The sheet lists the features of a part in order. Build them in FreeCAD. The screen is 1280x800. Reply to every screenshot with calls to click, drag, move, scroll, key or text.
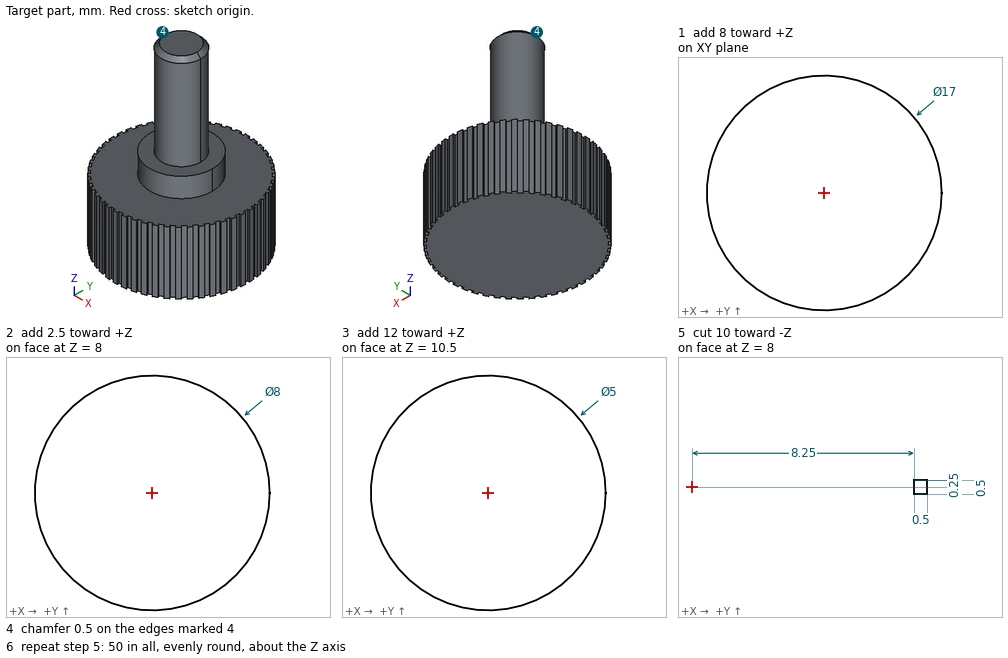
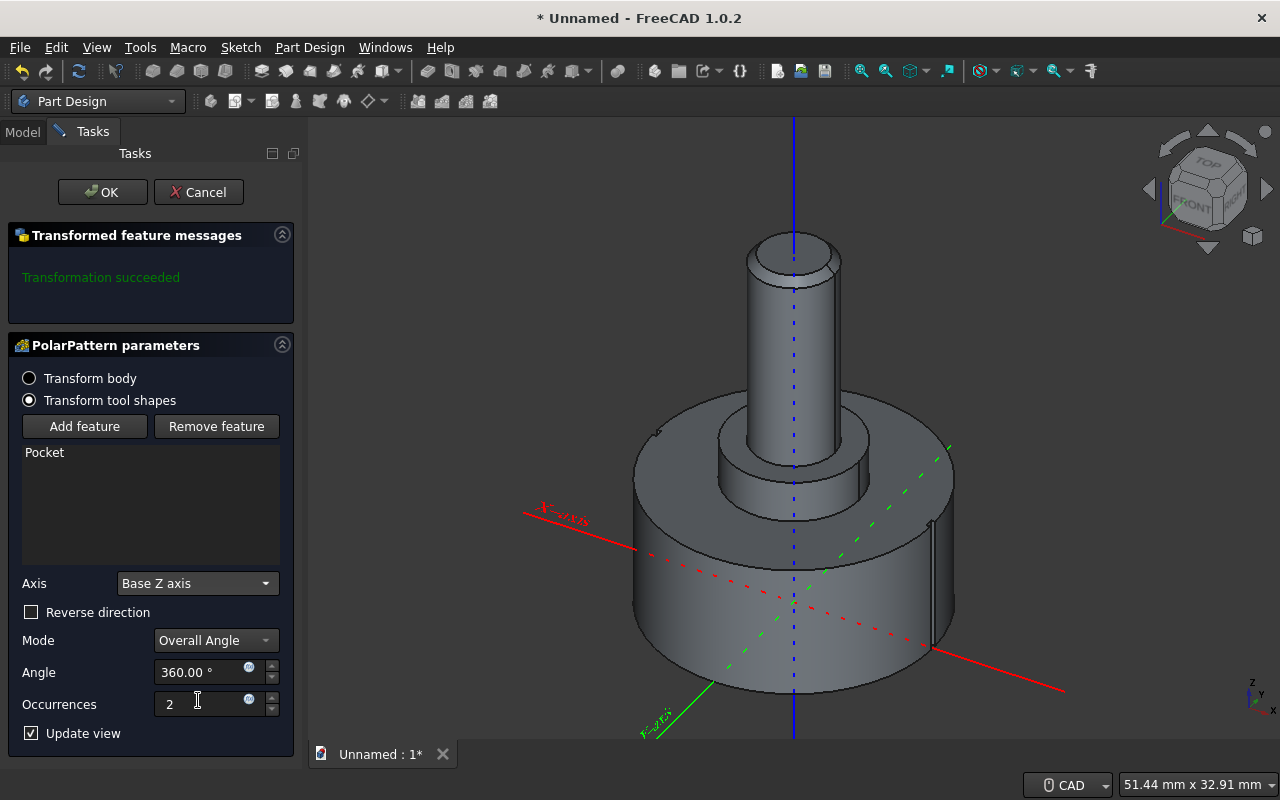
triple_click(209, 704)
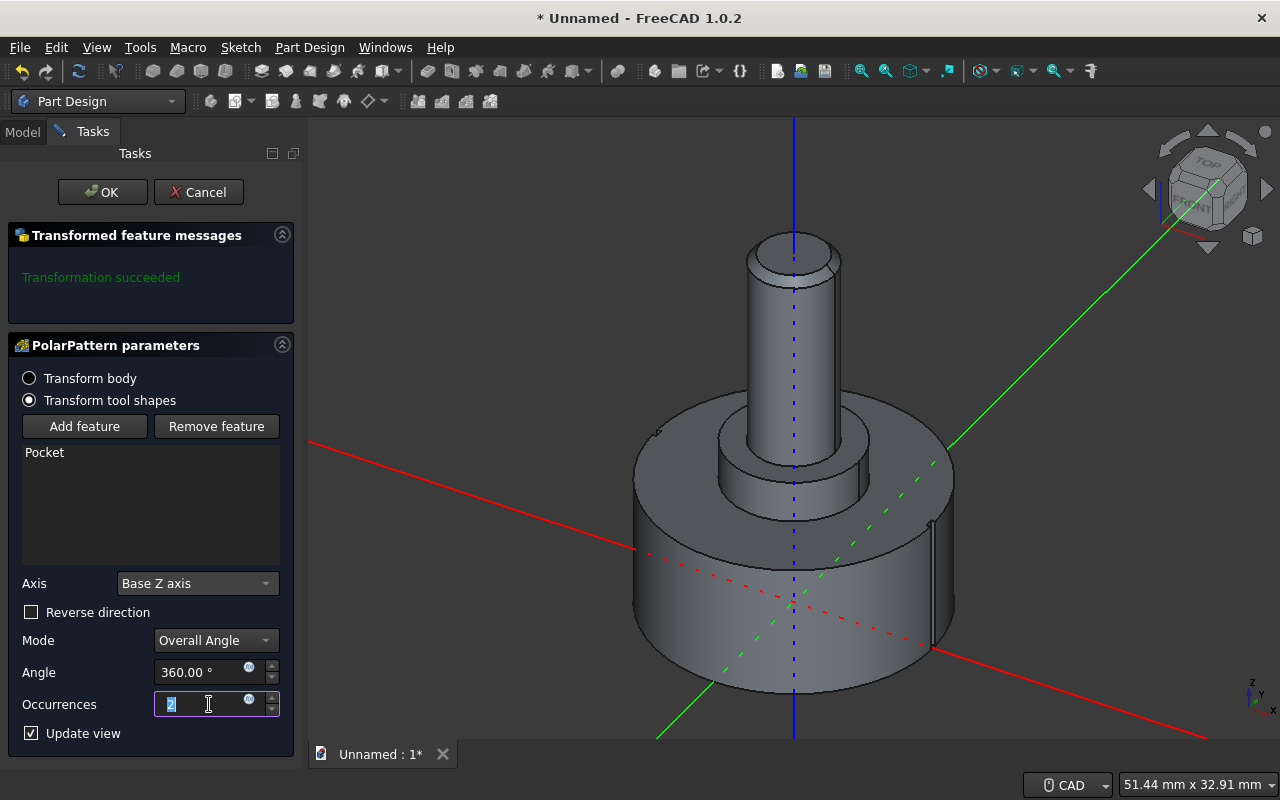
text(50)
key(Tab)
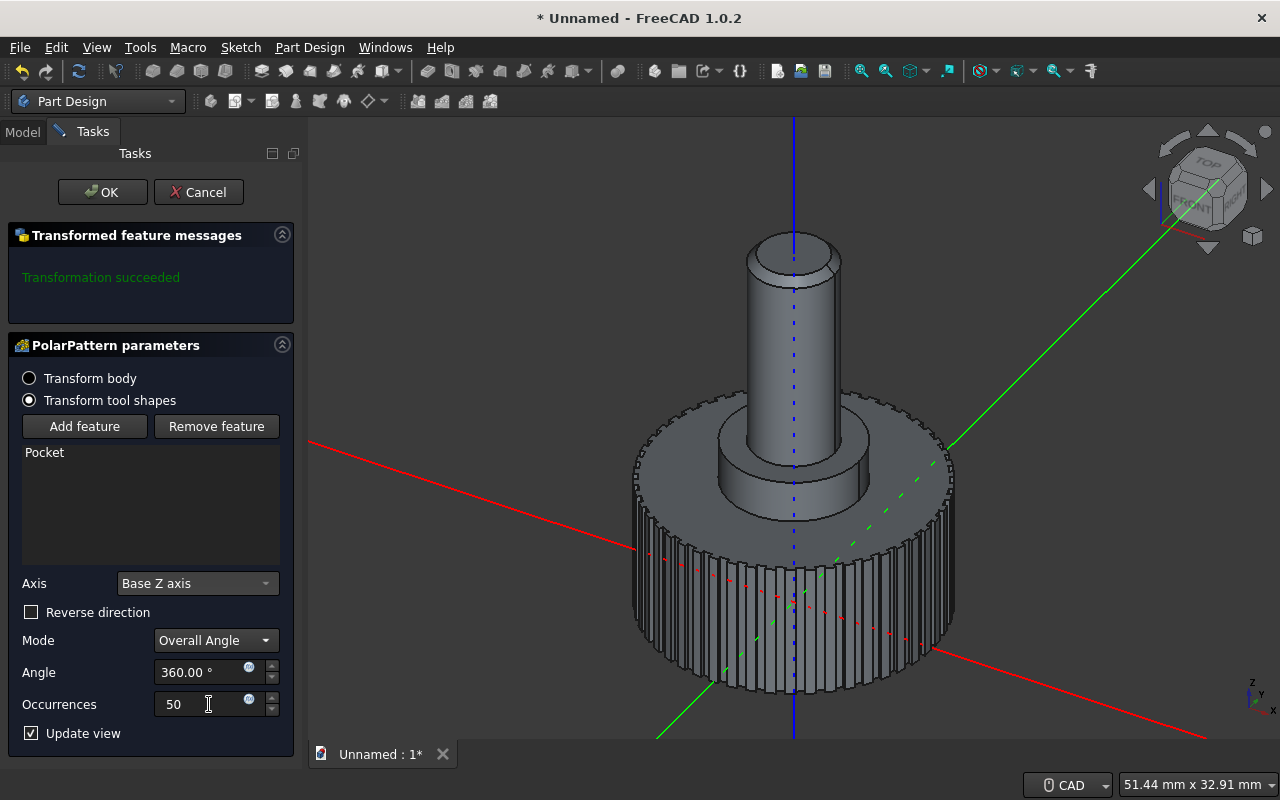
click(103, 192)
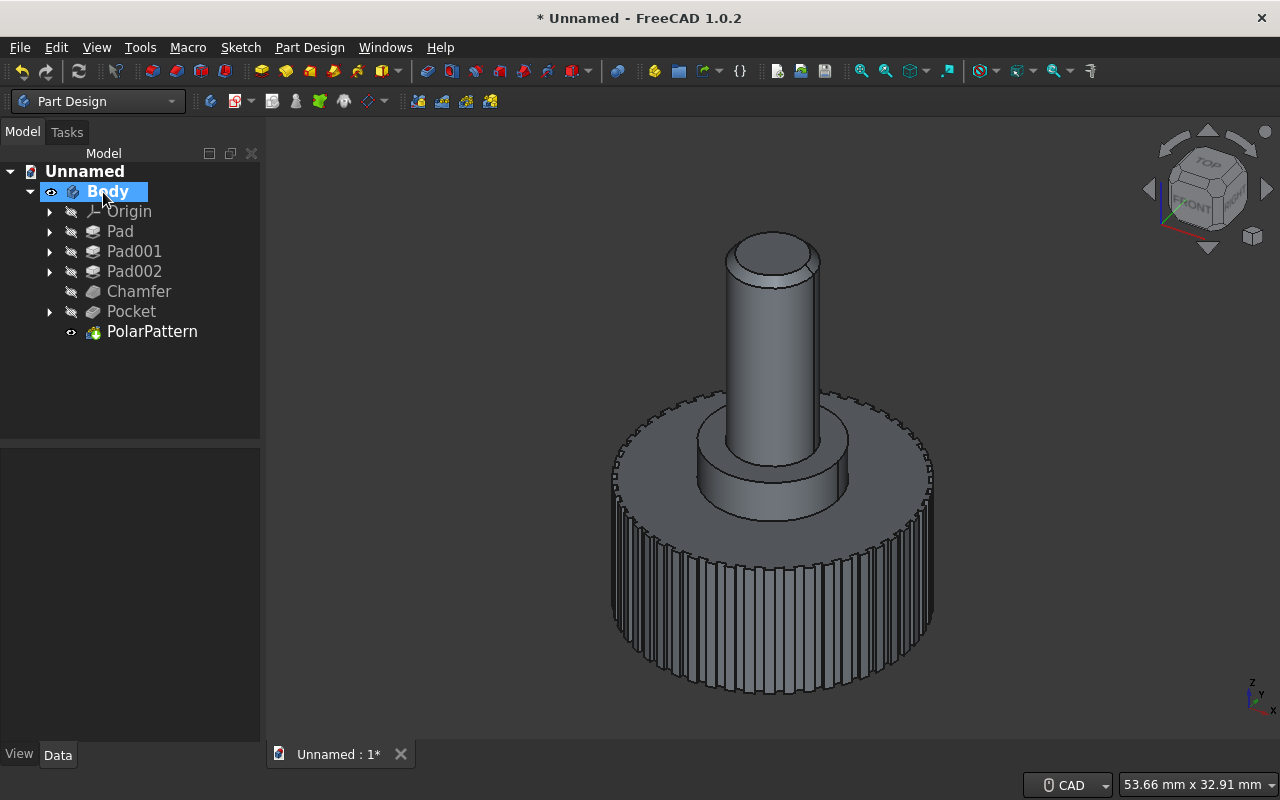
key(0)